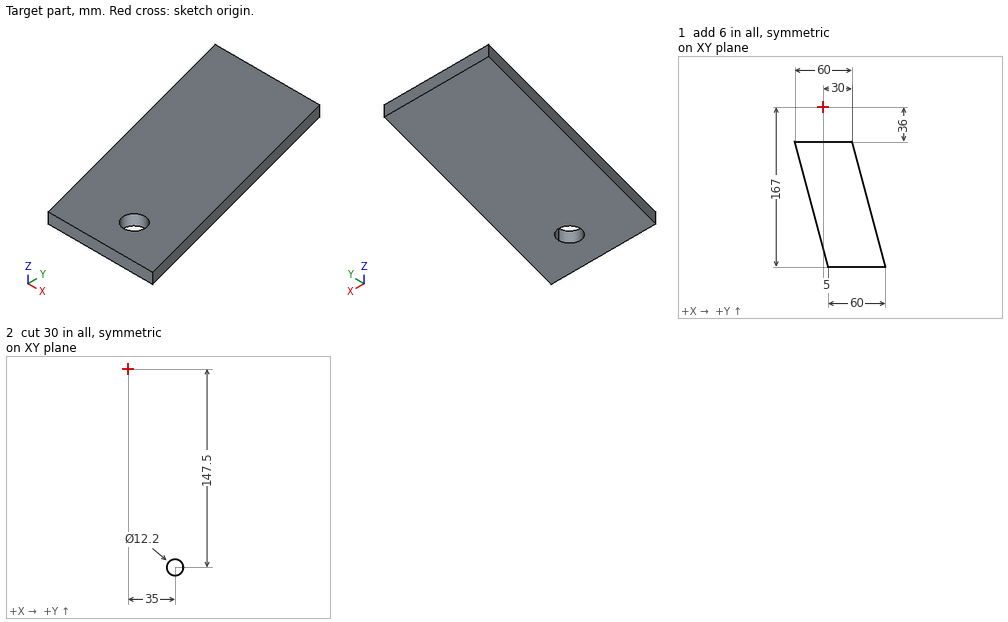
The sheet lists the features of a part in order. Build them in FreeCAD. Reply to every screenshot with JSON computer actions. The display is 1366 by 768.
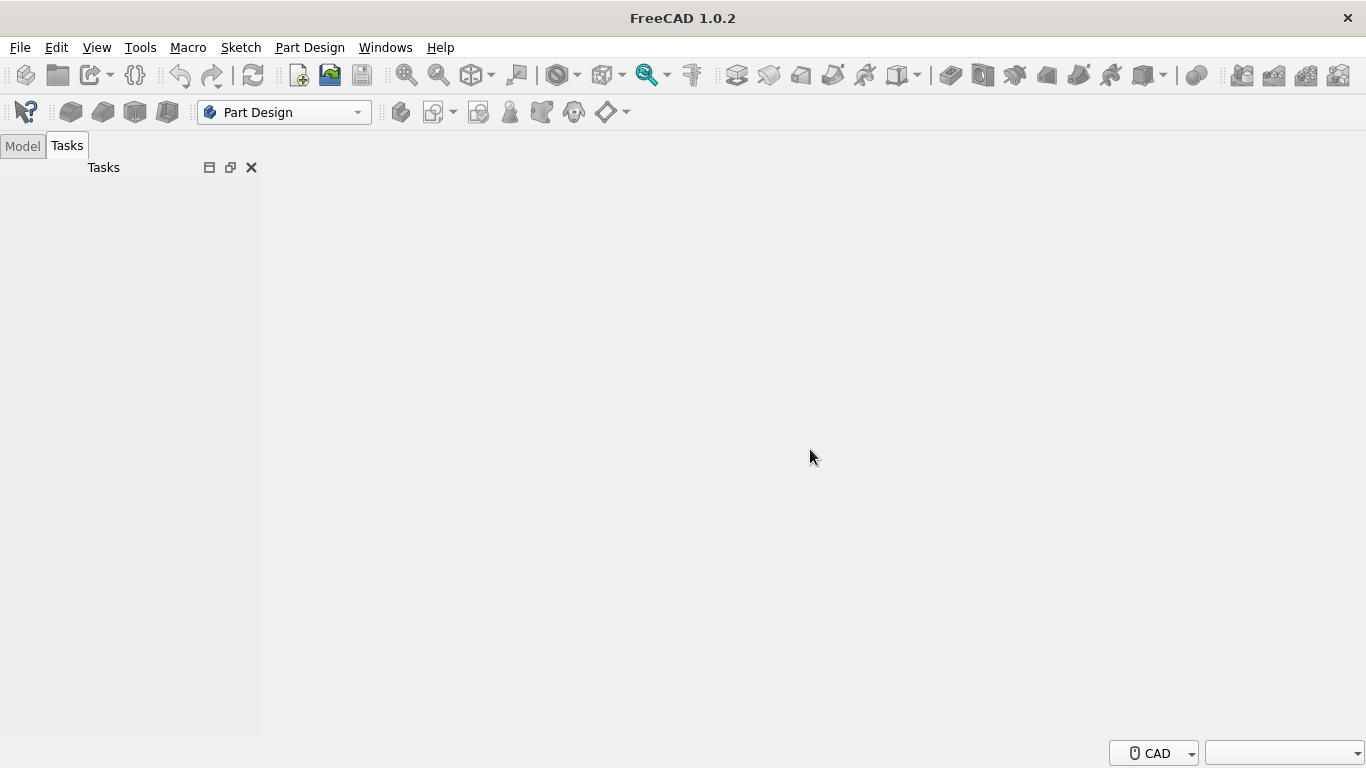
{"action": "left_click", "coordinate": [298, 76]}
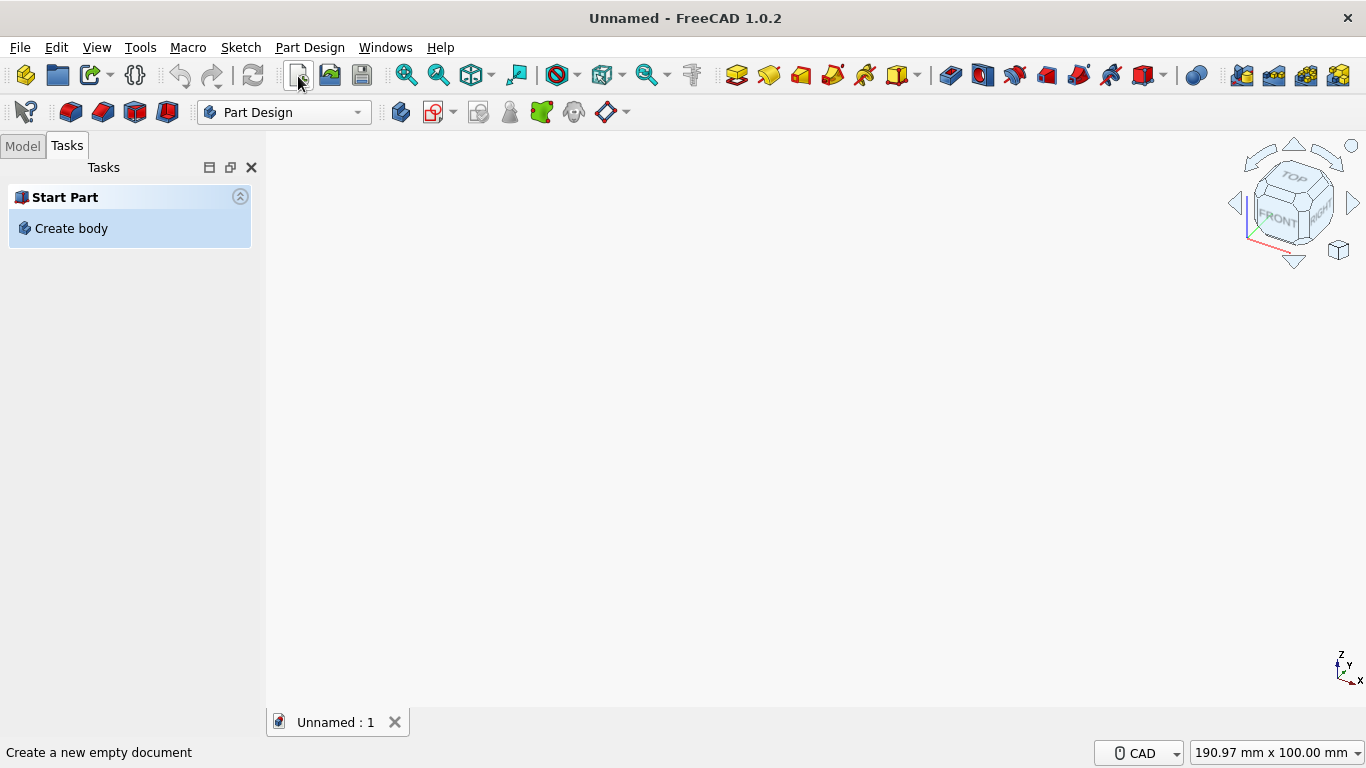
{"action": "left_click", "coordinate": [434, 112]}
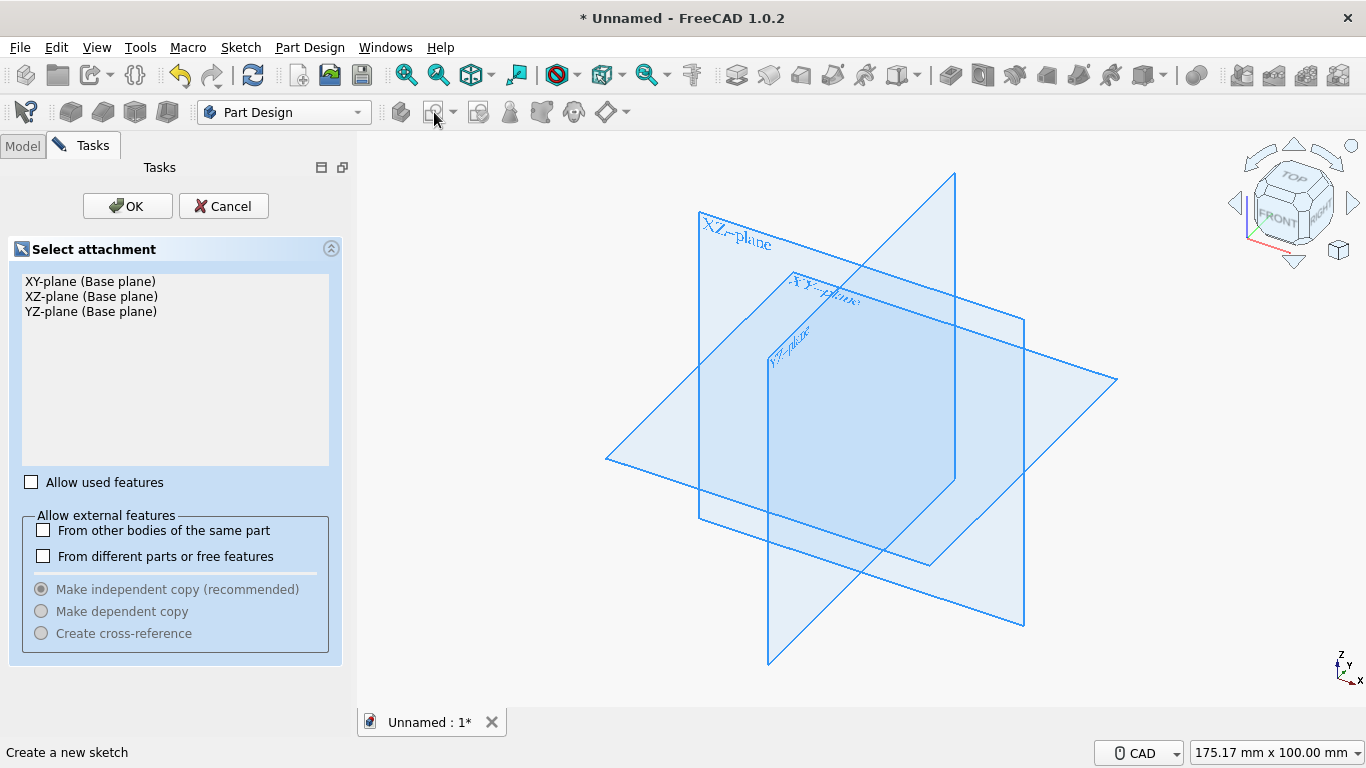
{"action": "left_click", "coordinate": [82, 282]}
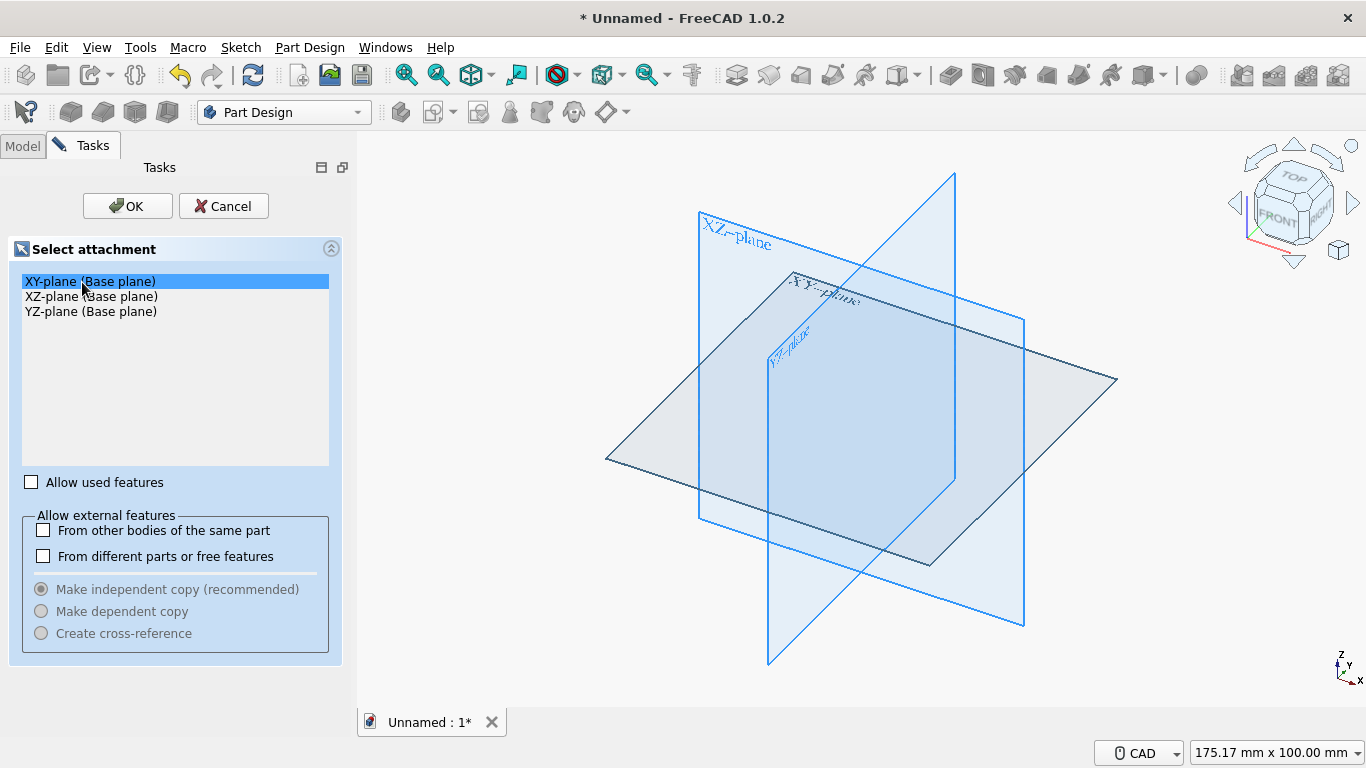
{"action": "left_click", "coordinate": [128, 206]}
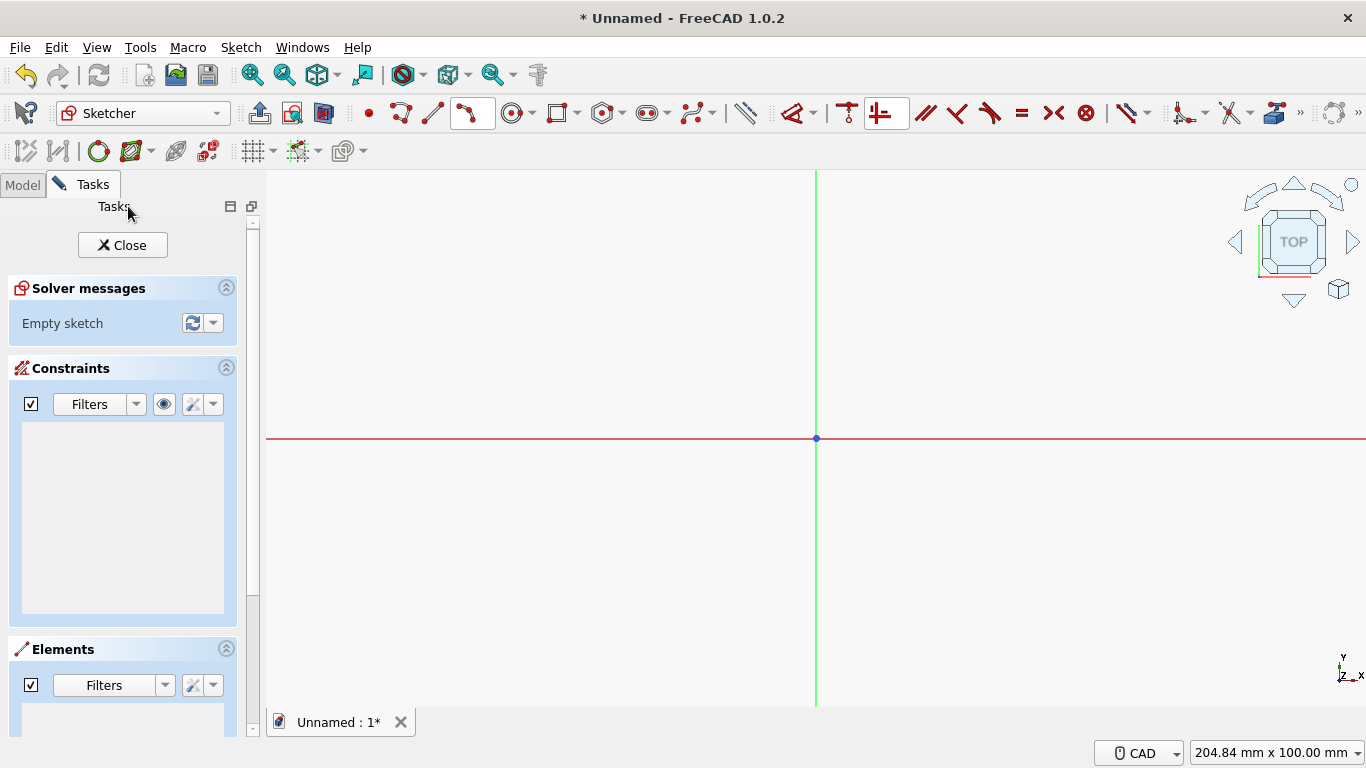
{"action": "scroll", "coordinate": [653, 198], "scroll_direction": "down", "scroll_amount": 5}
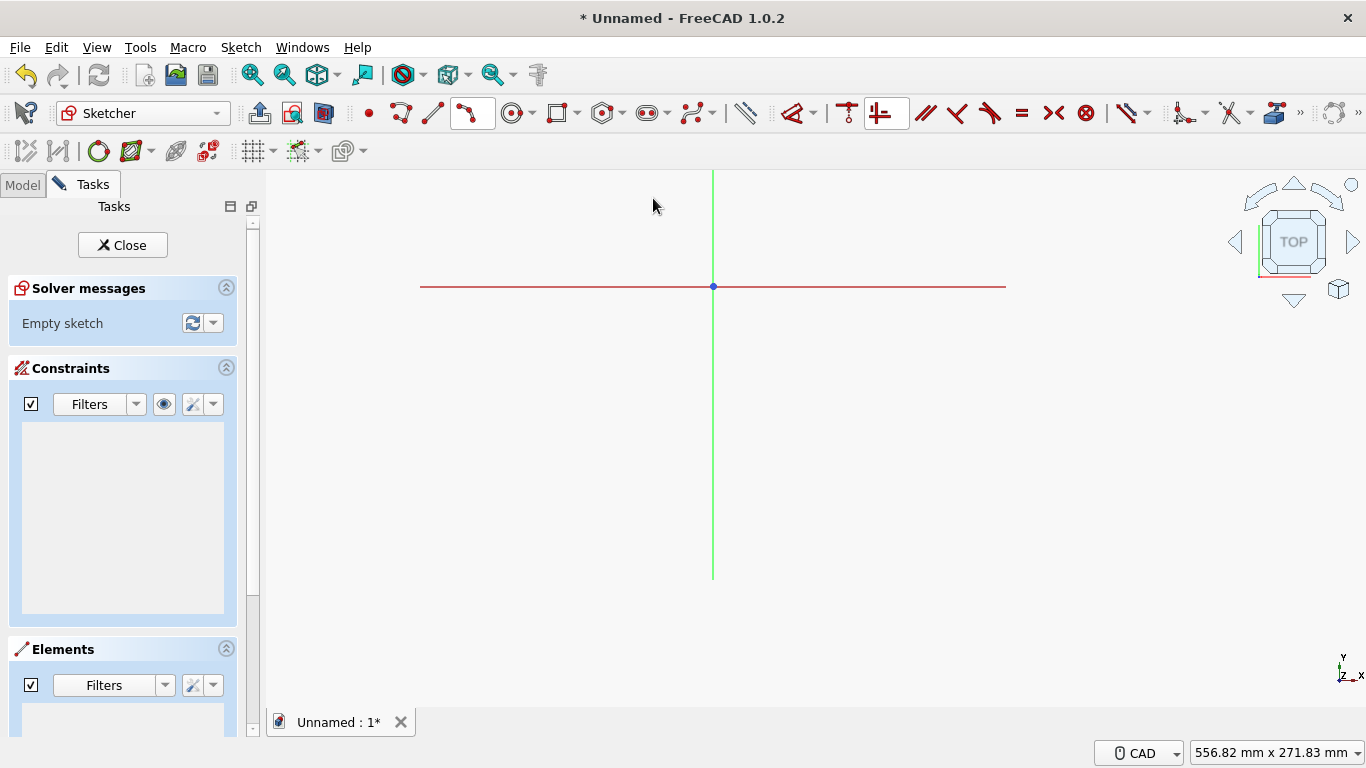
{"action": "left_click", "coordinate": [402, 114]}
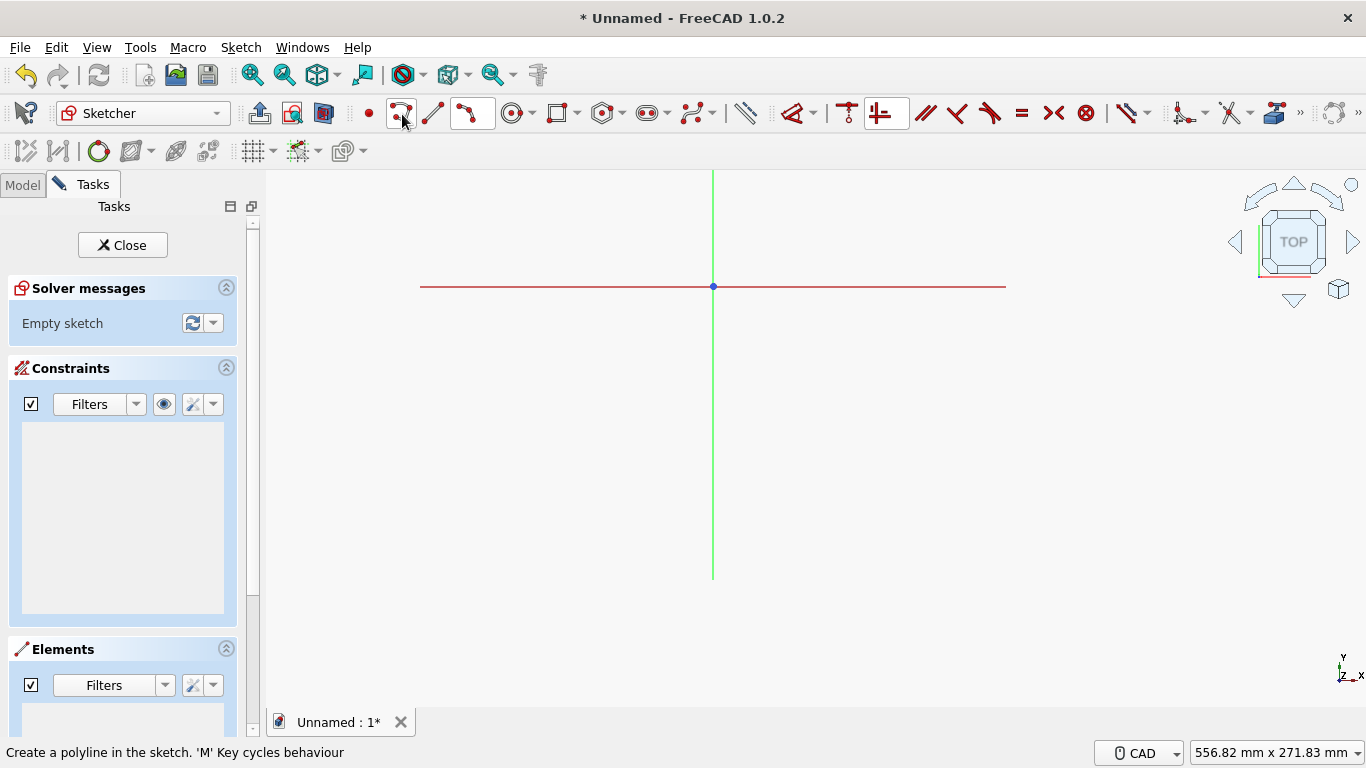
{"action": "left_click", "coordinate": [772, 358]}
{"action": "left_click", "coordinate": [654, 358]}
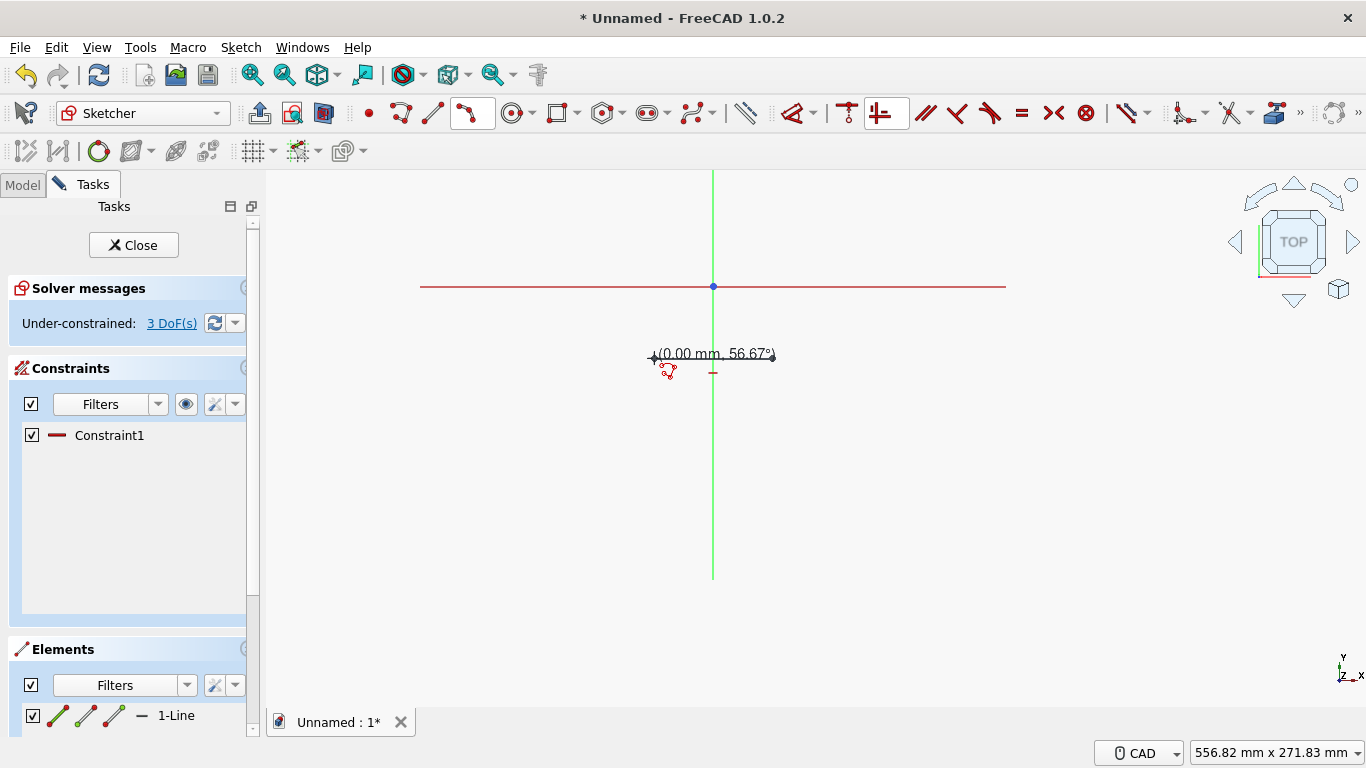
{"action": "scroll", "coordinate": [723, 616], "scroll_direction": "up", "scroll_amount": 3}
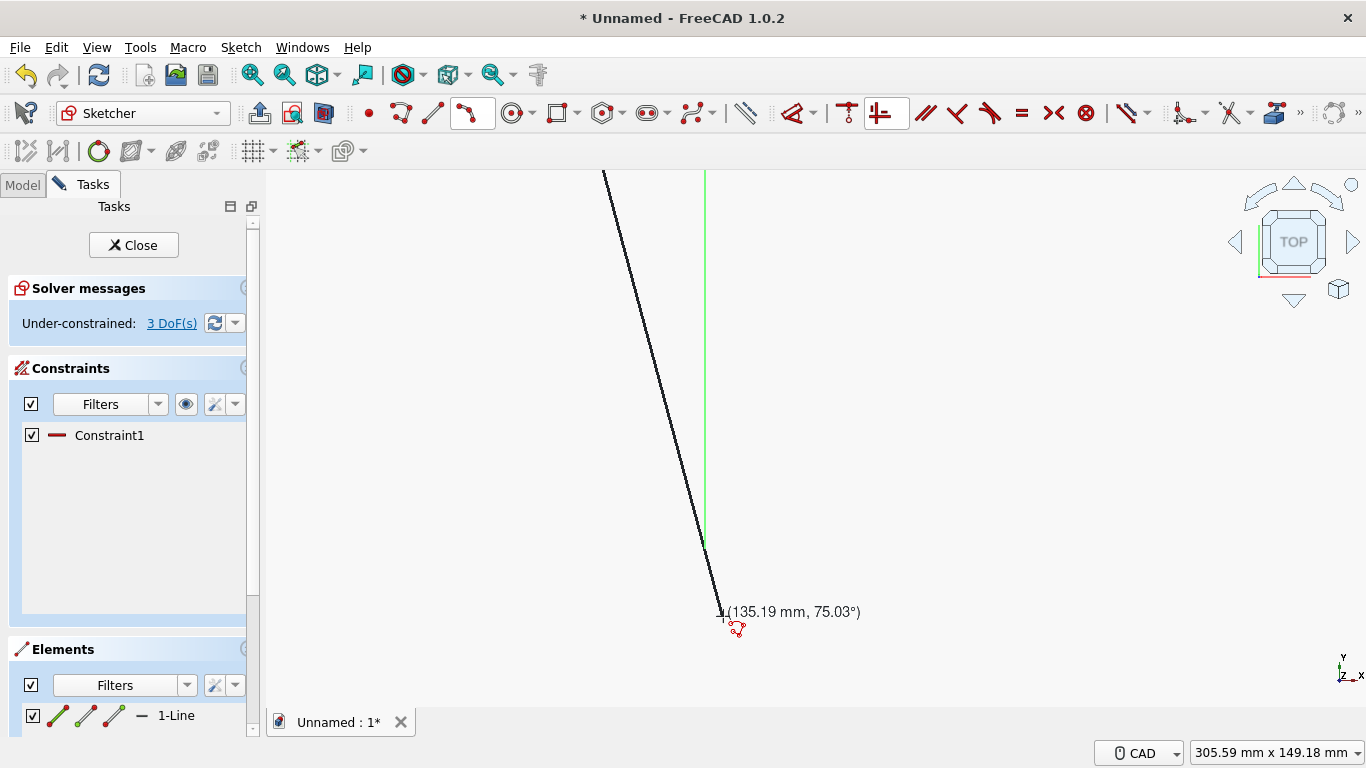
{"action": "left_click", "coordinate": [723, 616]}
{"action": "left_click", "coordinate": [939, 616]}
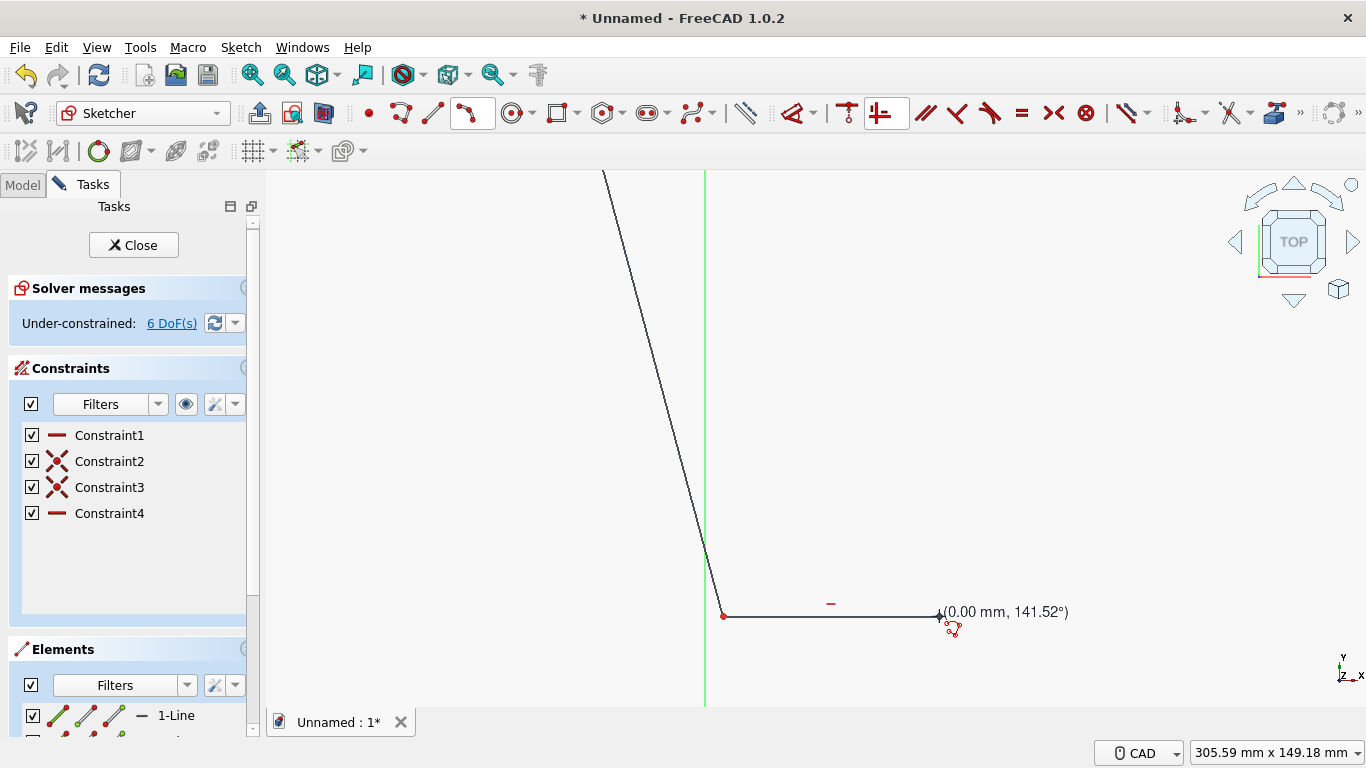
{"action": "scroll", "coordinate": [723, 588], "scroll_direction": "down", "scroll_amount": 3}